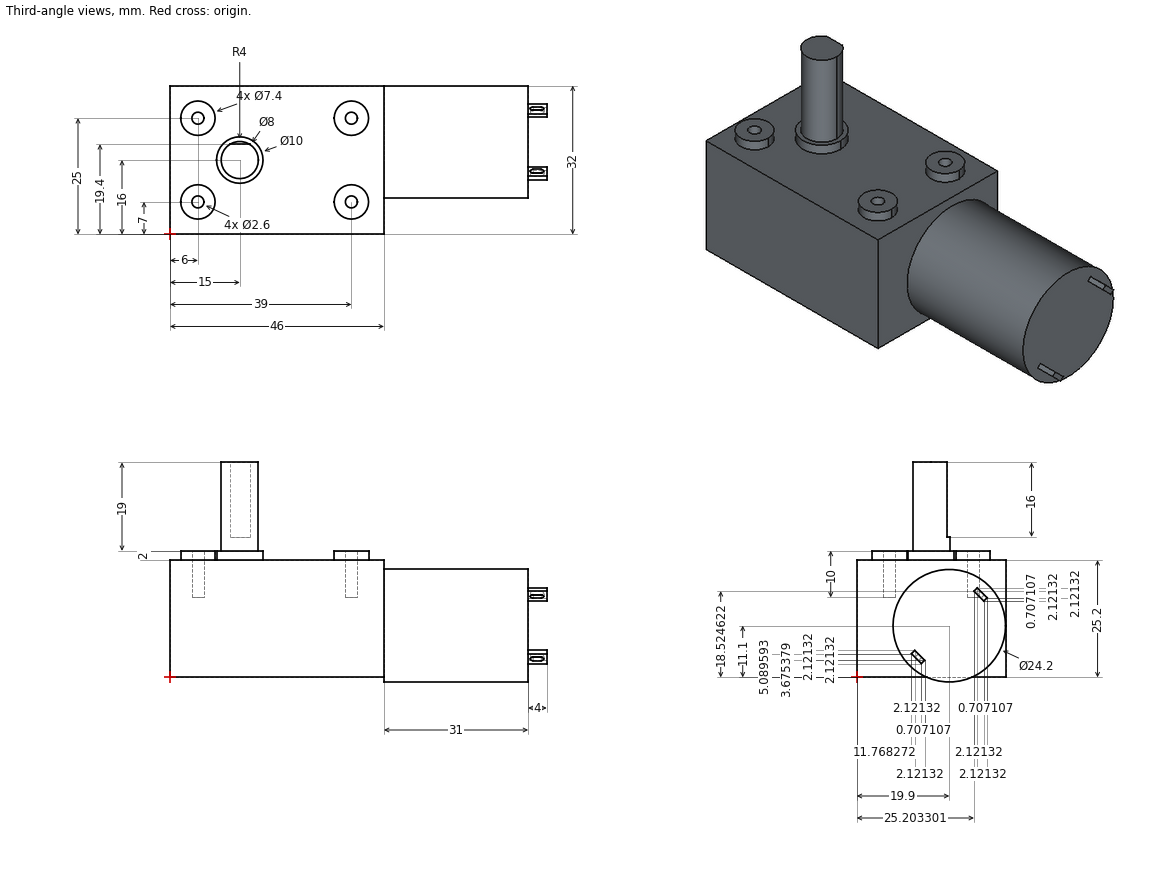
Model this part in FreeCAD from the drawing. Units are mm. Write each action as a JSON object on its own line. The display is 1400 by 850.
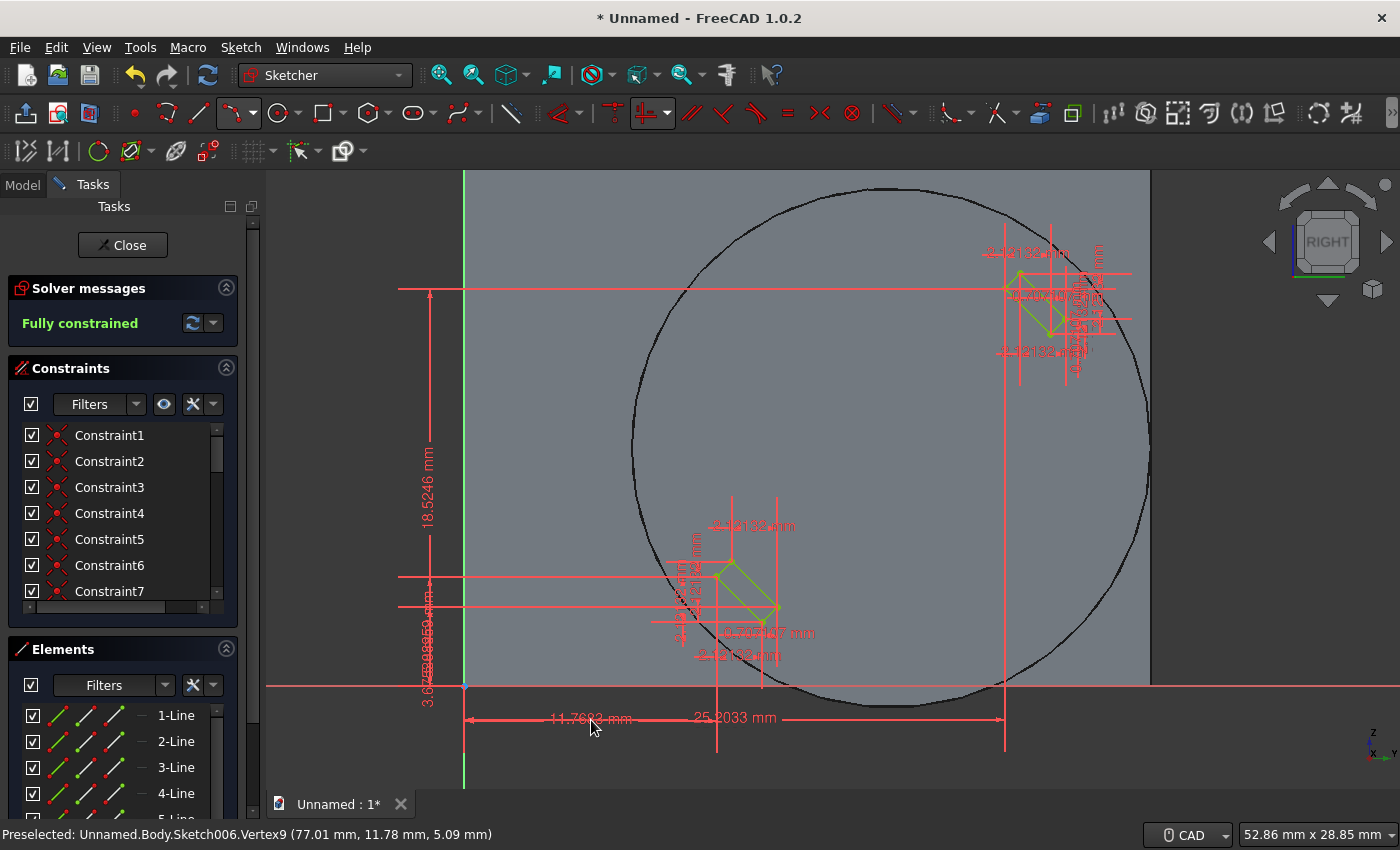
{"action": "left_click", "coordinate": [123, 245]}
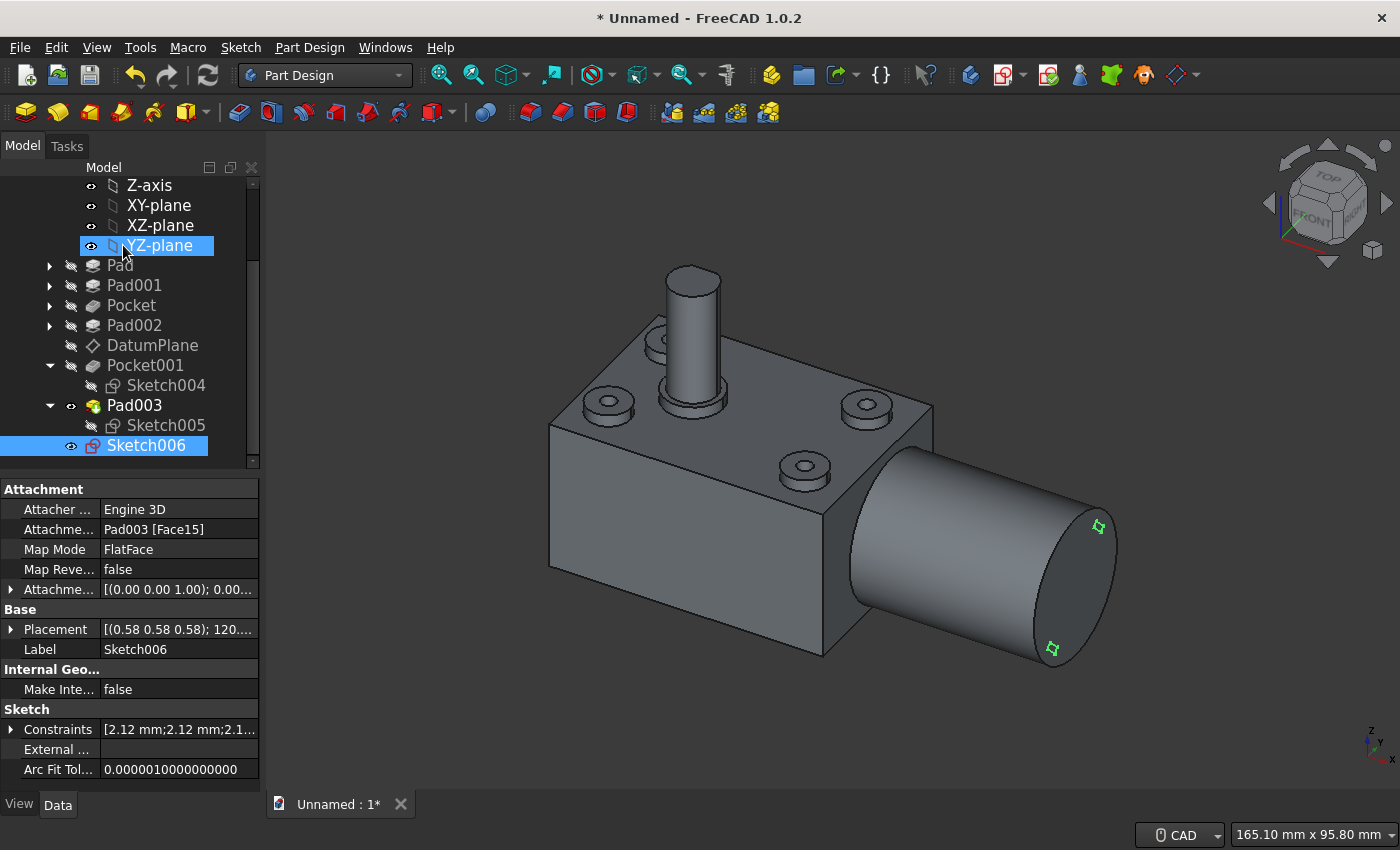
{"action": "left_click", "coordinate": [26, 112]}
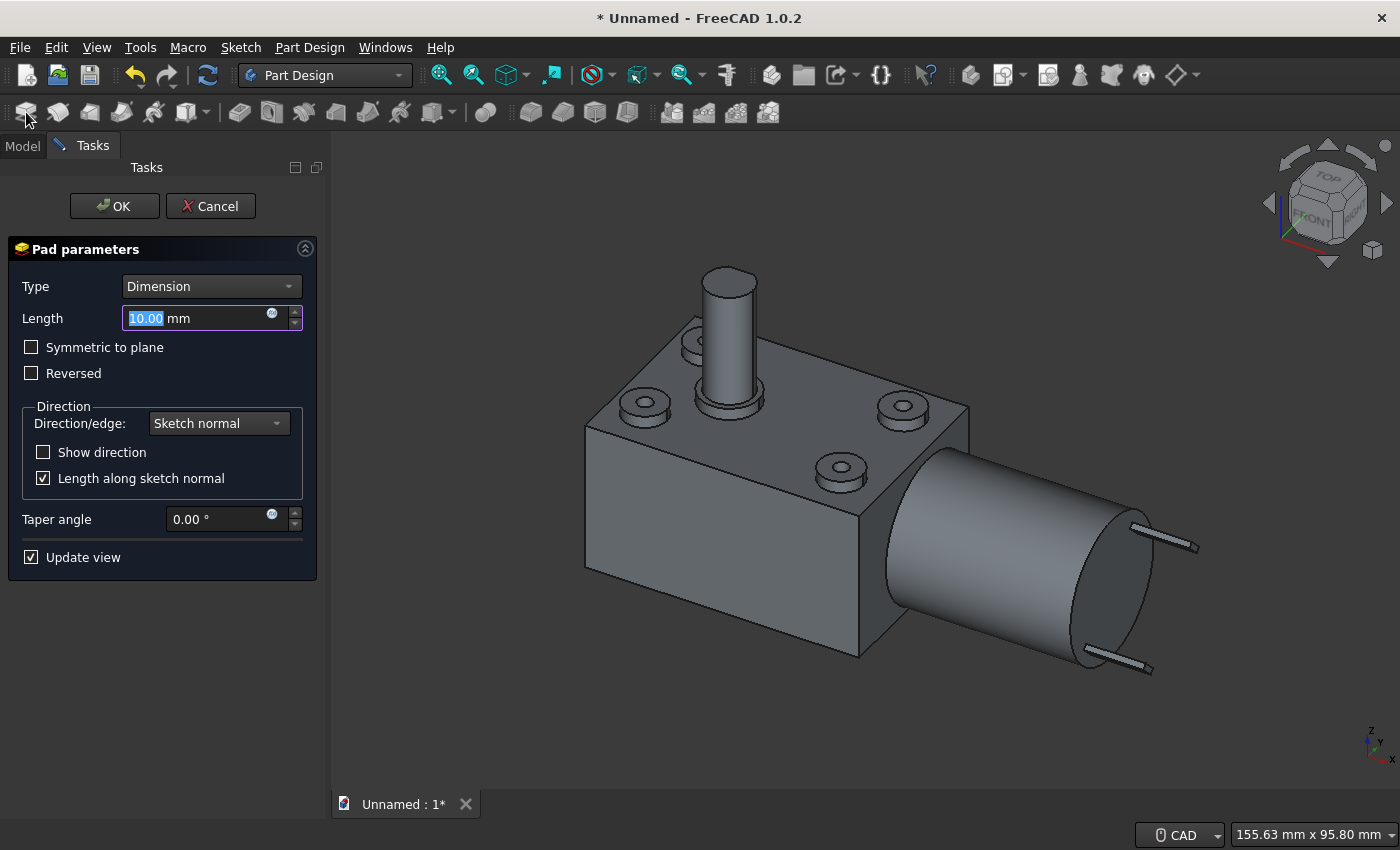
{"action": "type", "text": "4"}
{"action": "key", "text": "Tab"}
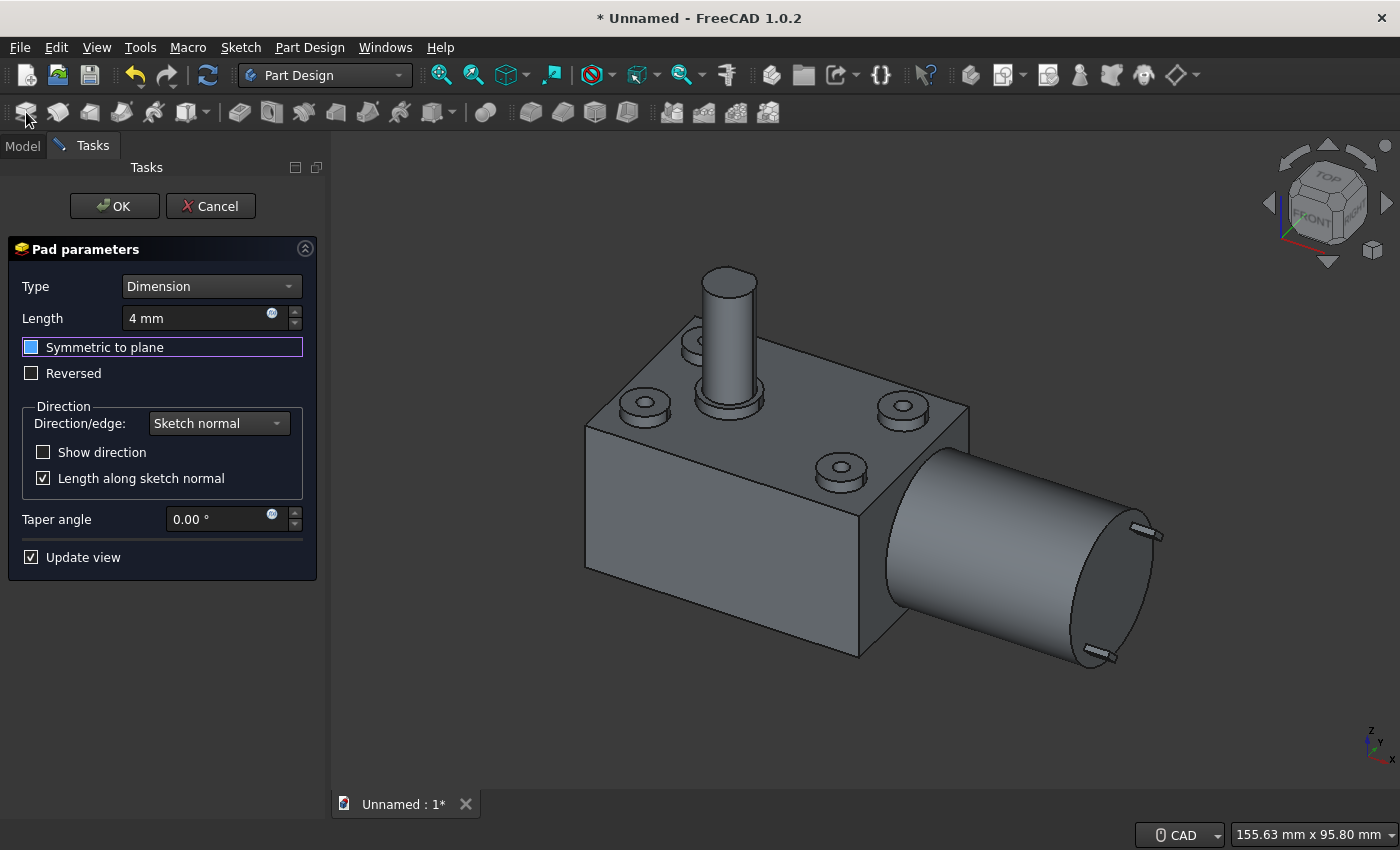
{"action": "left_click", "coordinate": [115, 206]}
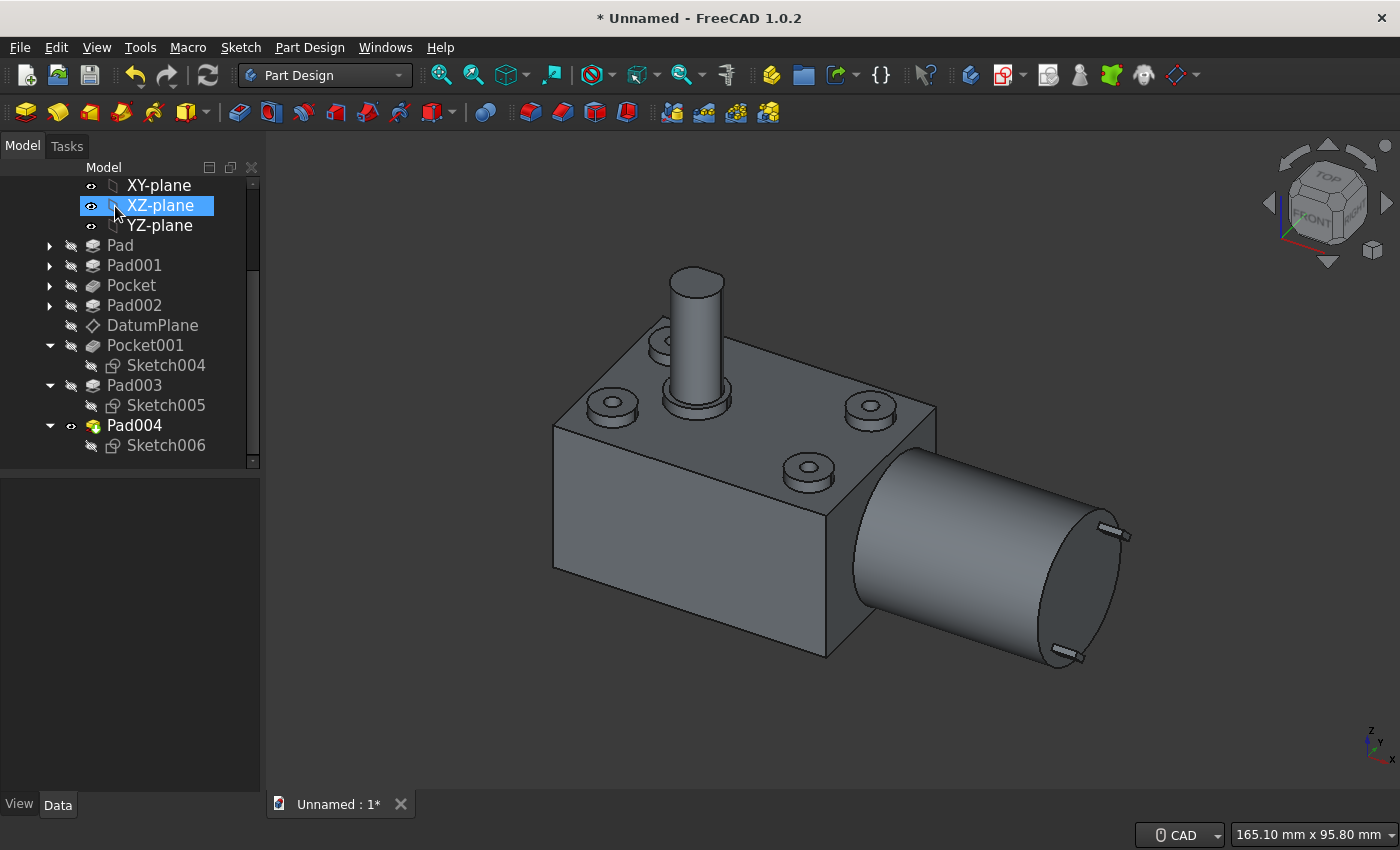
{"action": "key", "text": "2"}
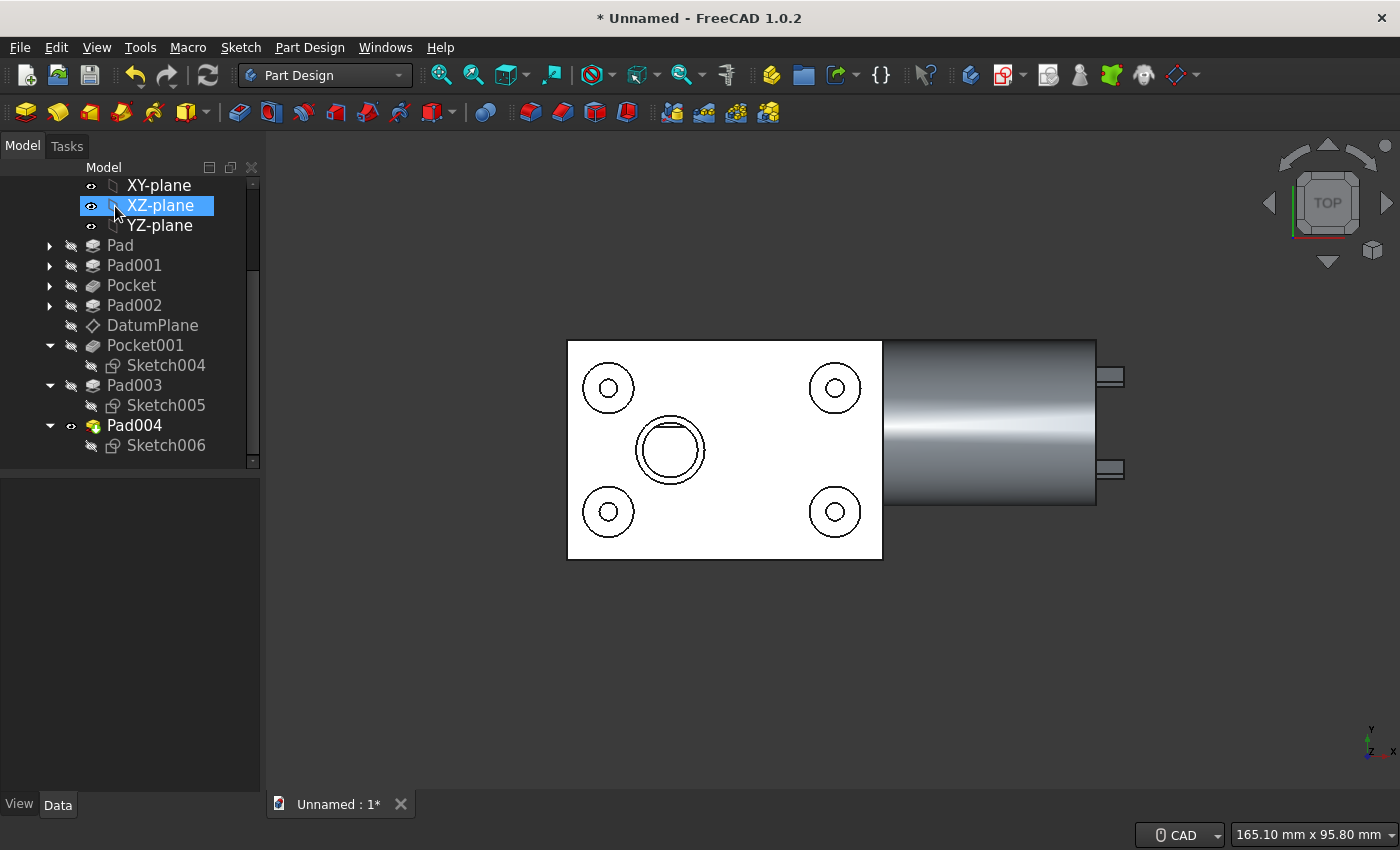
{"action": "left_click", "coordinate": [1114, 372]}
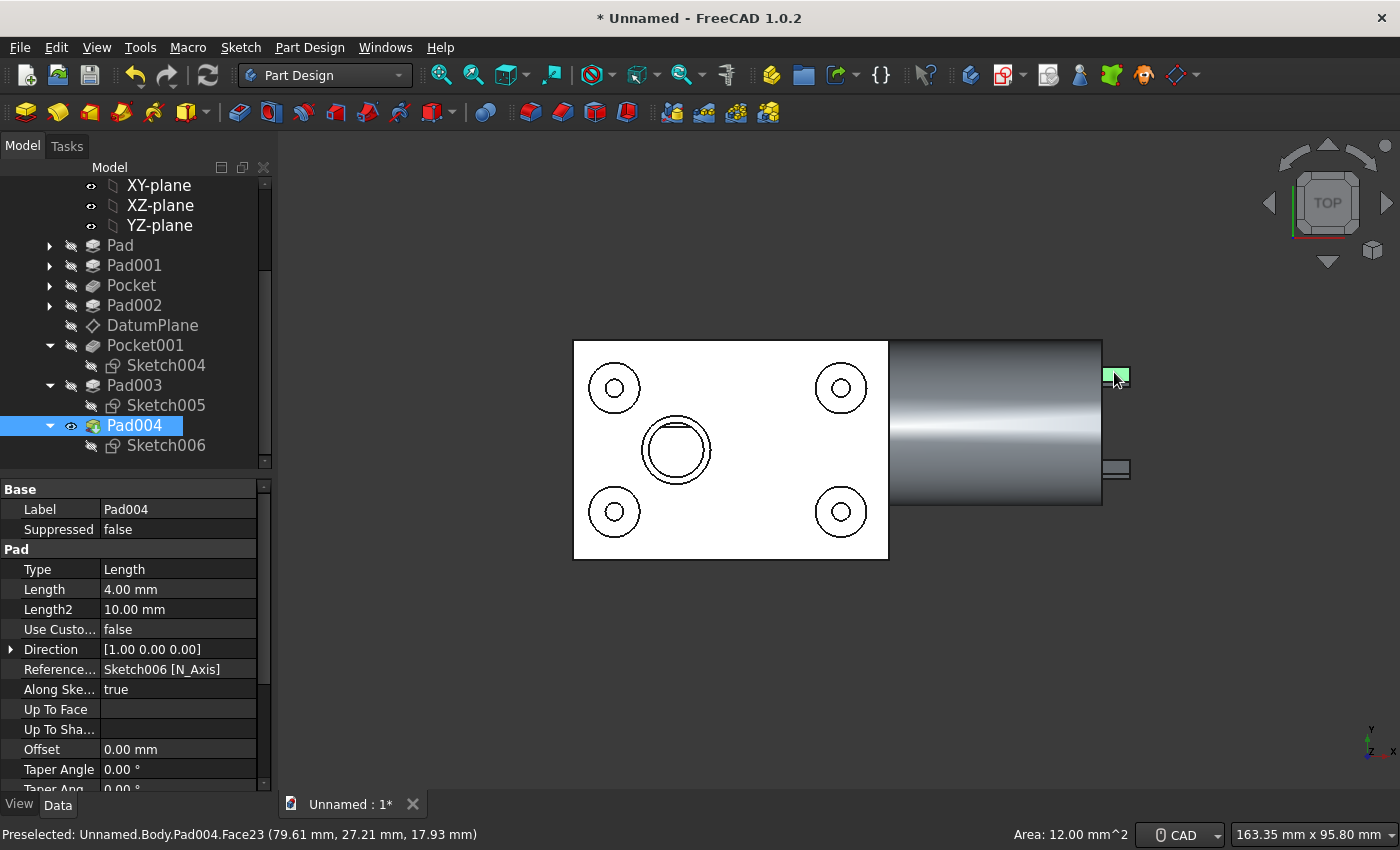
{"action": "left_click", "coordinate": [1004, 76]}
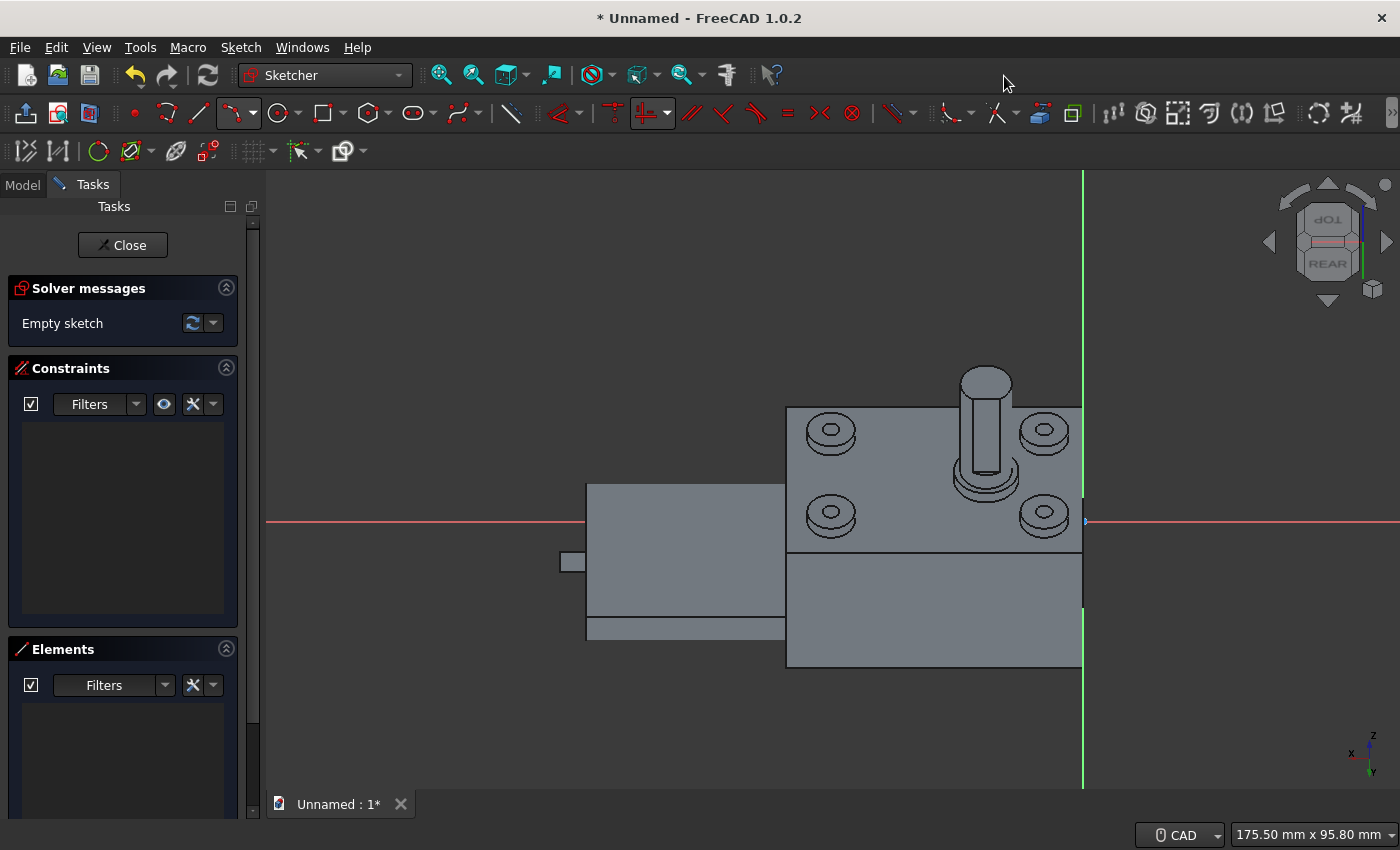
{"action": "left_click", "coordinate": [90, 114]}